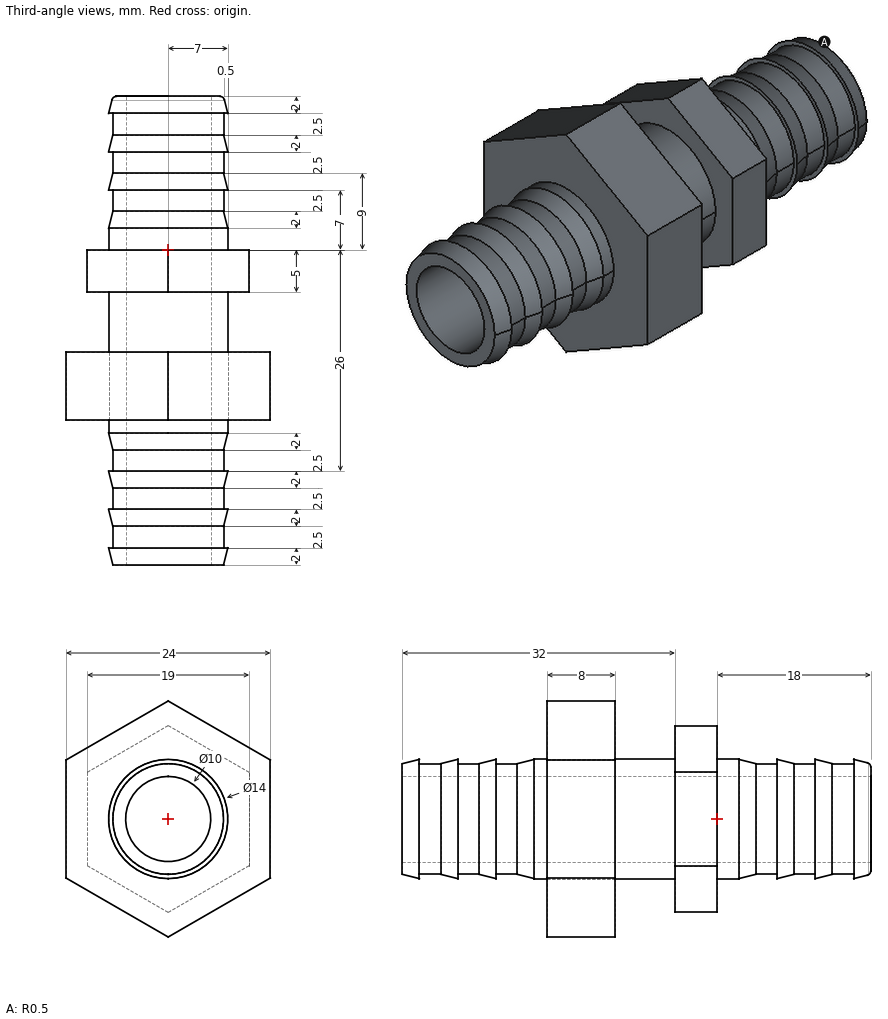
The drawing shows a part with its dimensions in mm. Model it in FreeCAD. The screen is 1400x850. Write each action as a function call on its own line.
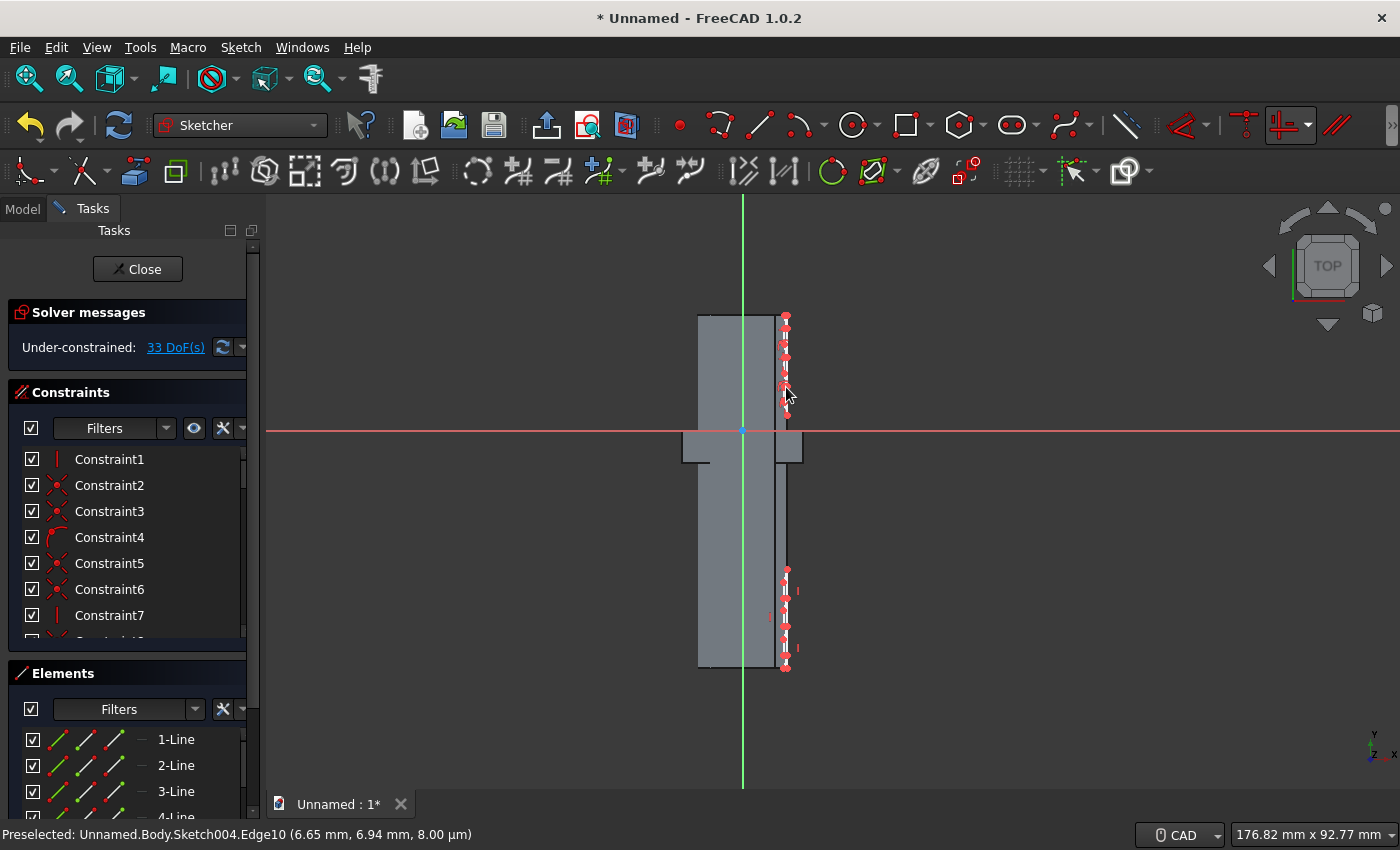
scroll(785, 599, up, 13)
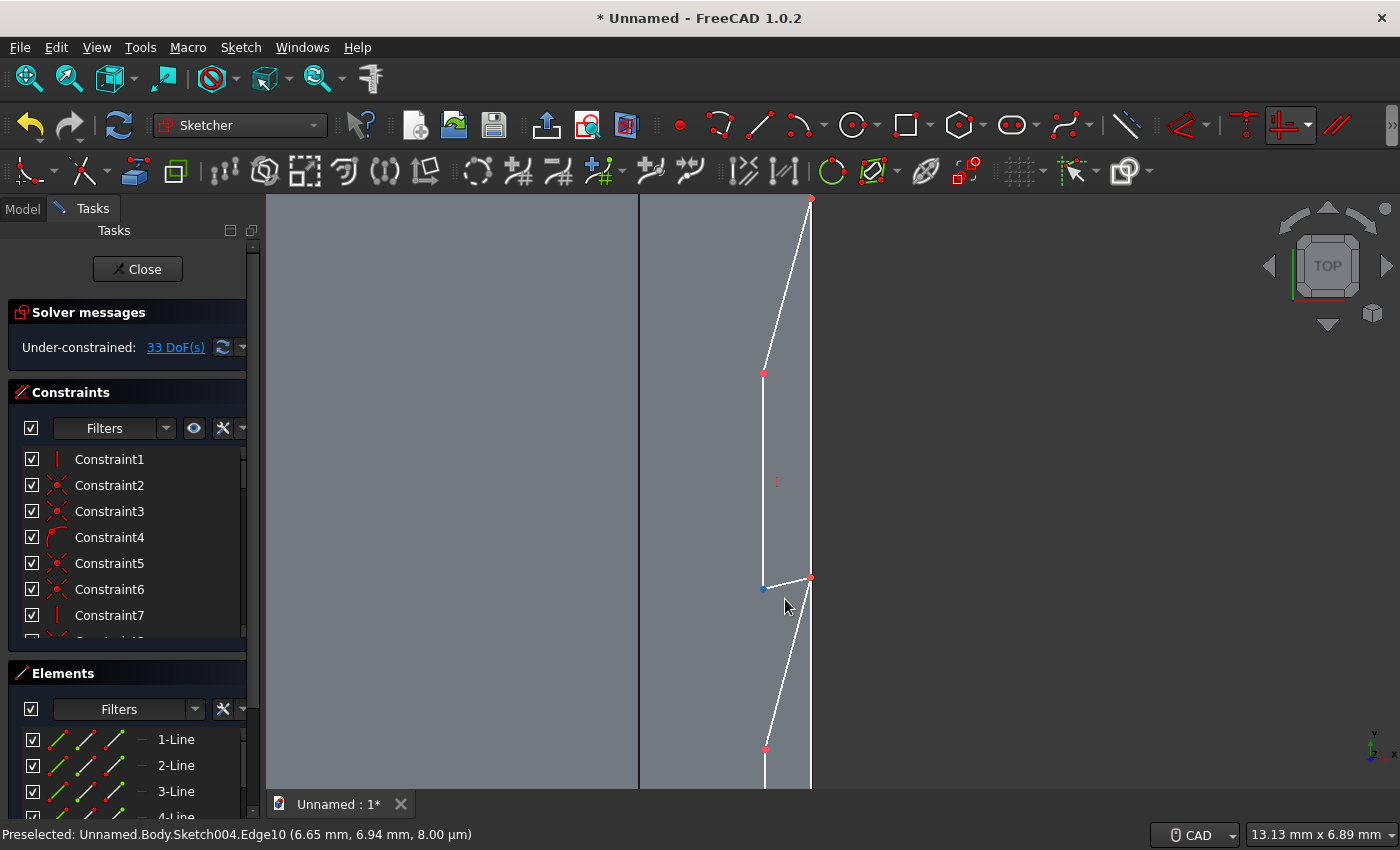
click(777, 586)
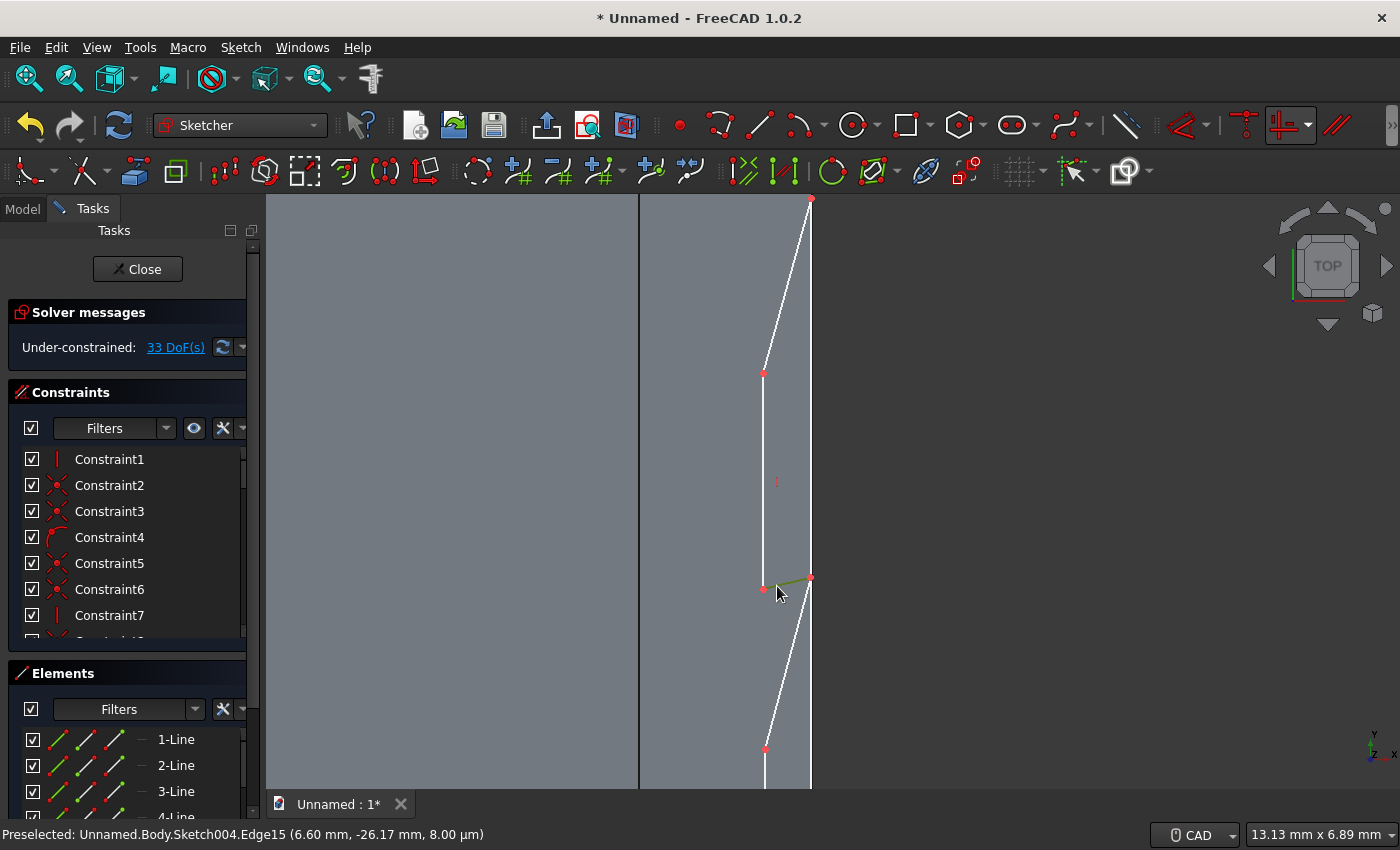
click(1310, 126)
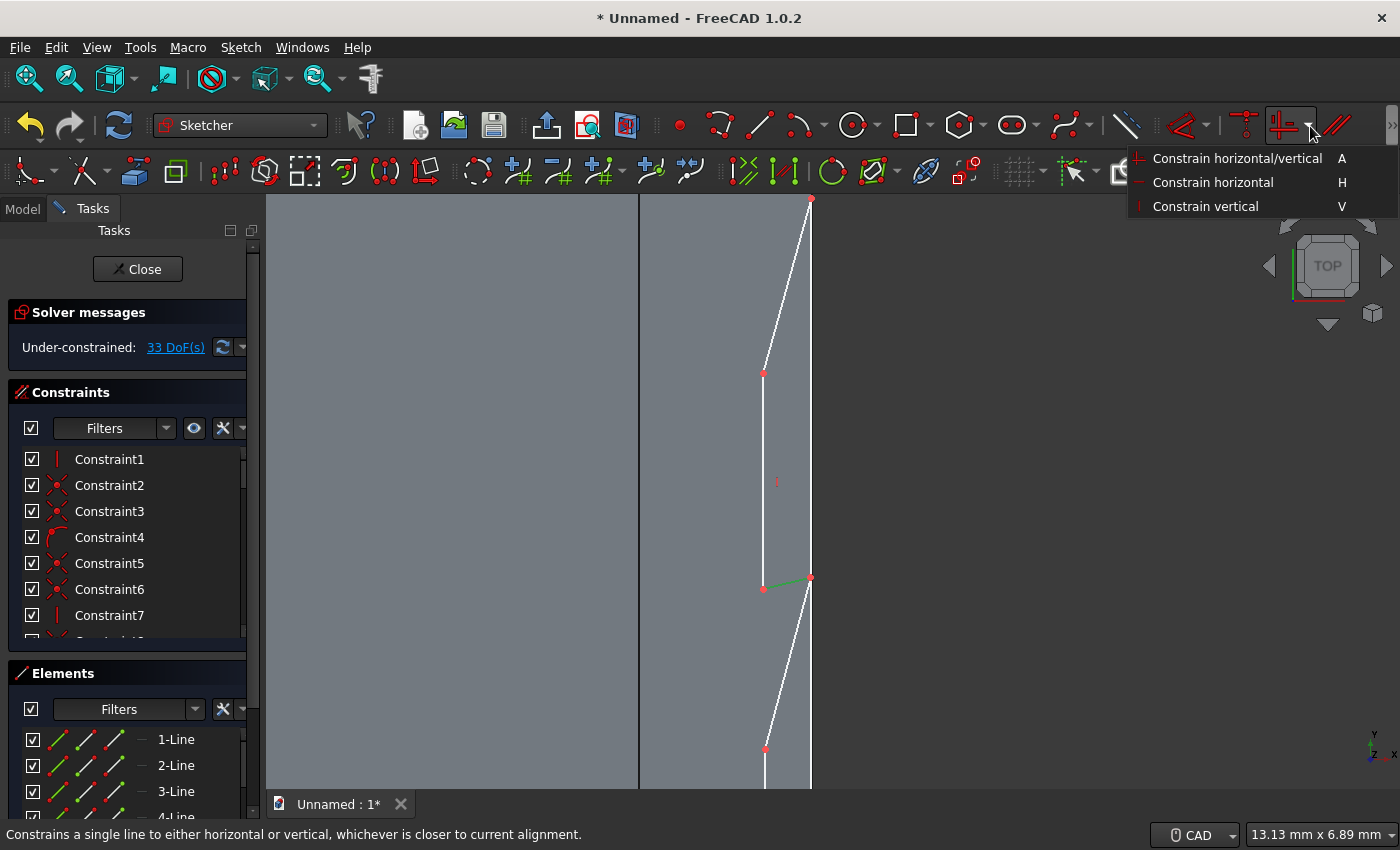
click(1263, 182)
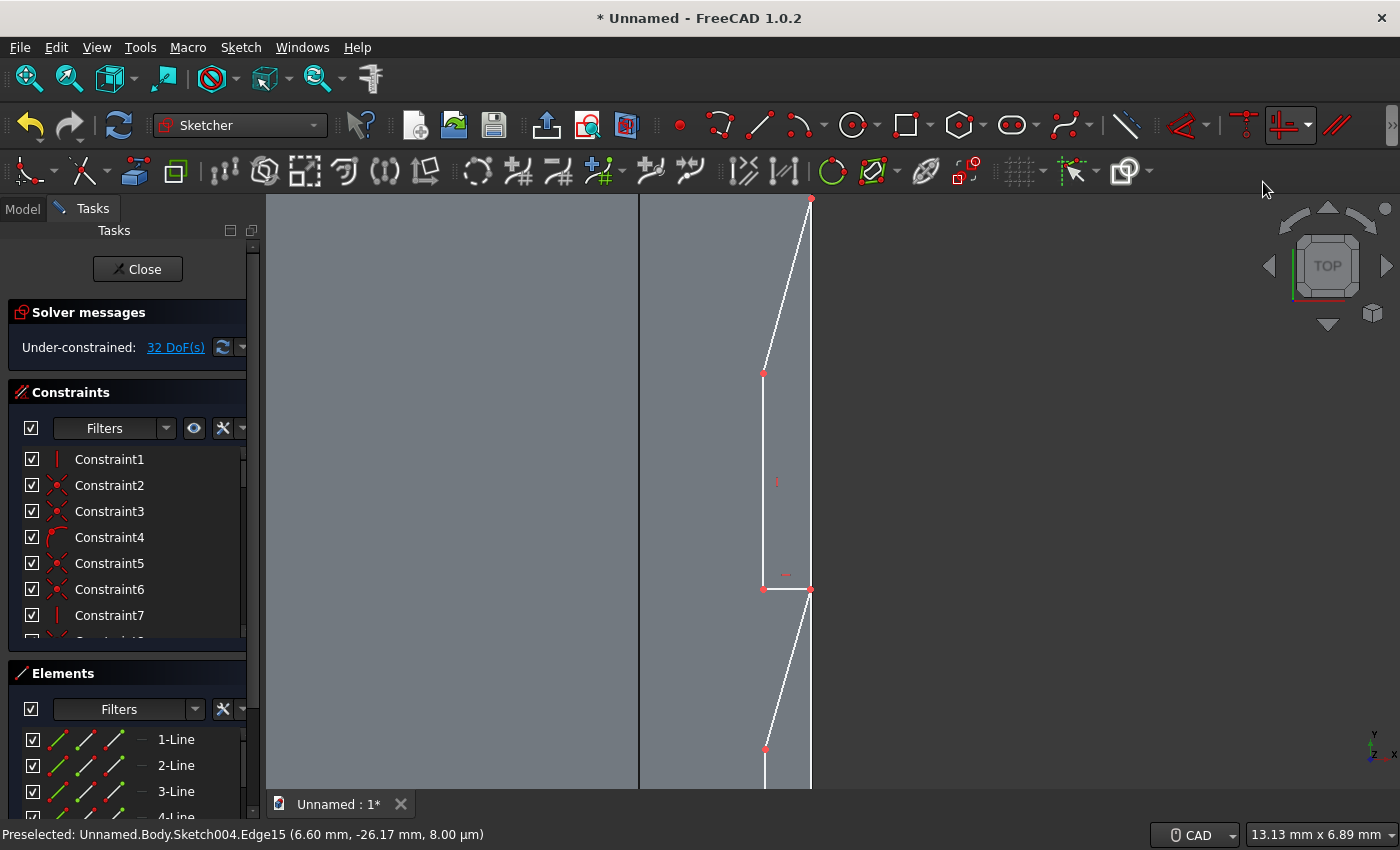
scroll(785, 599, down, 13)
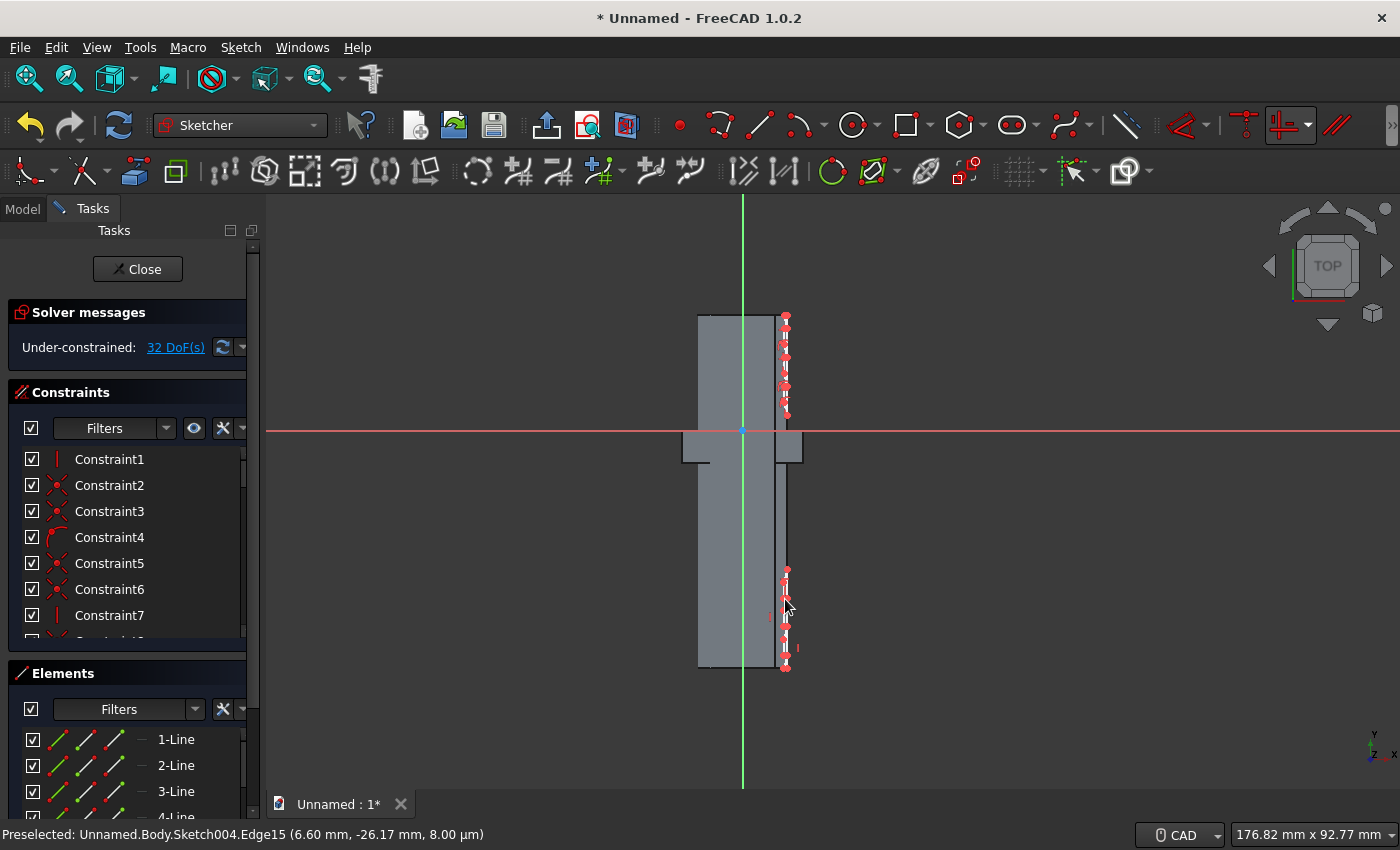
scroll(785, 627, up, 14)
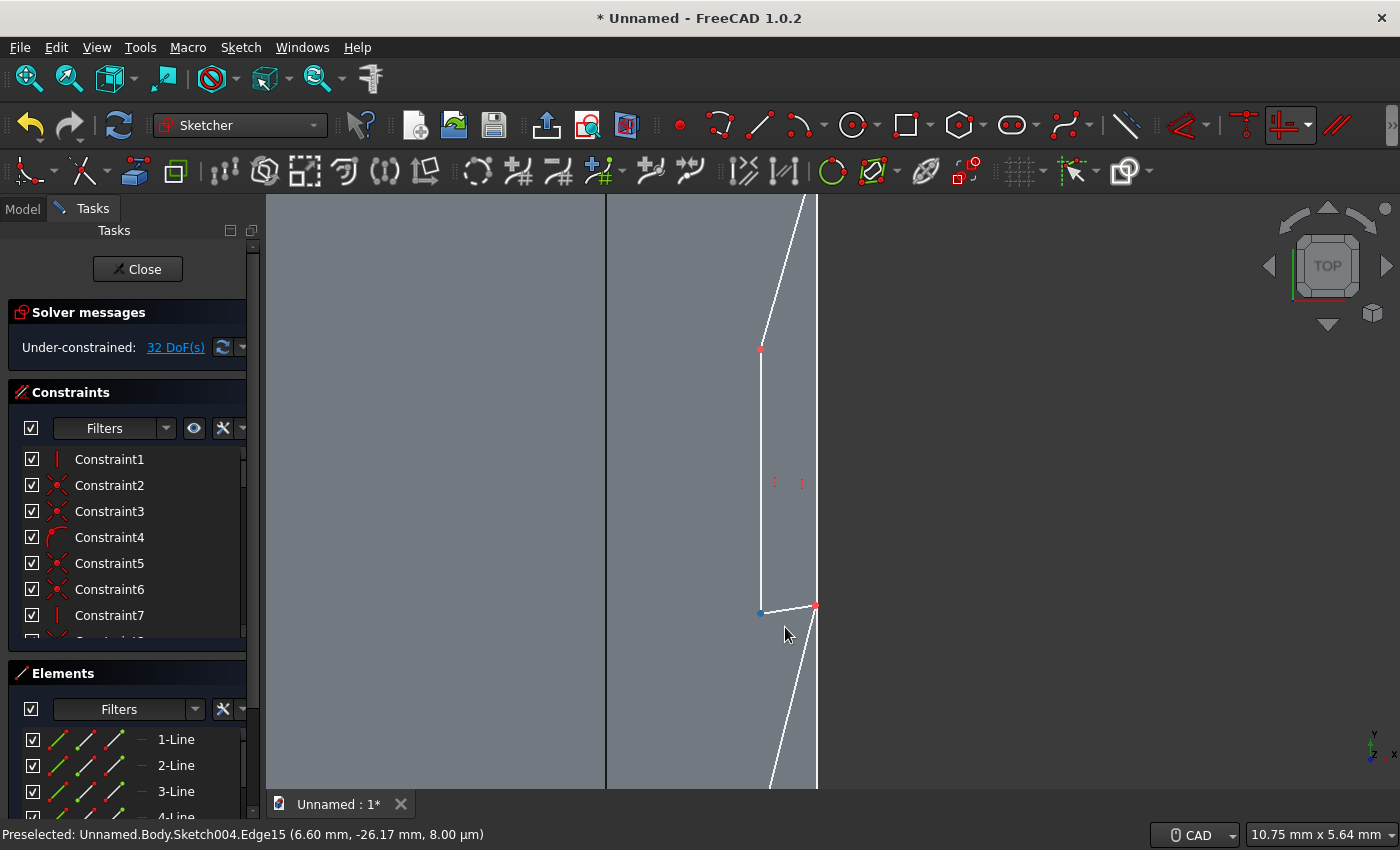
click(777, 611)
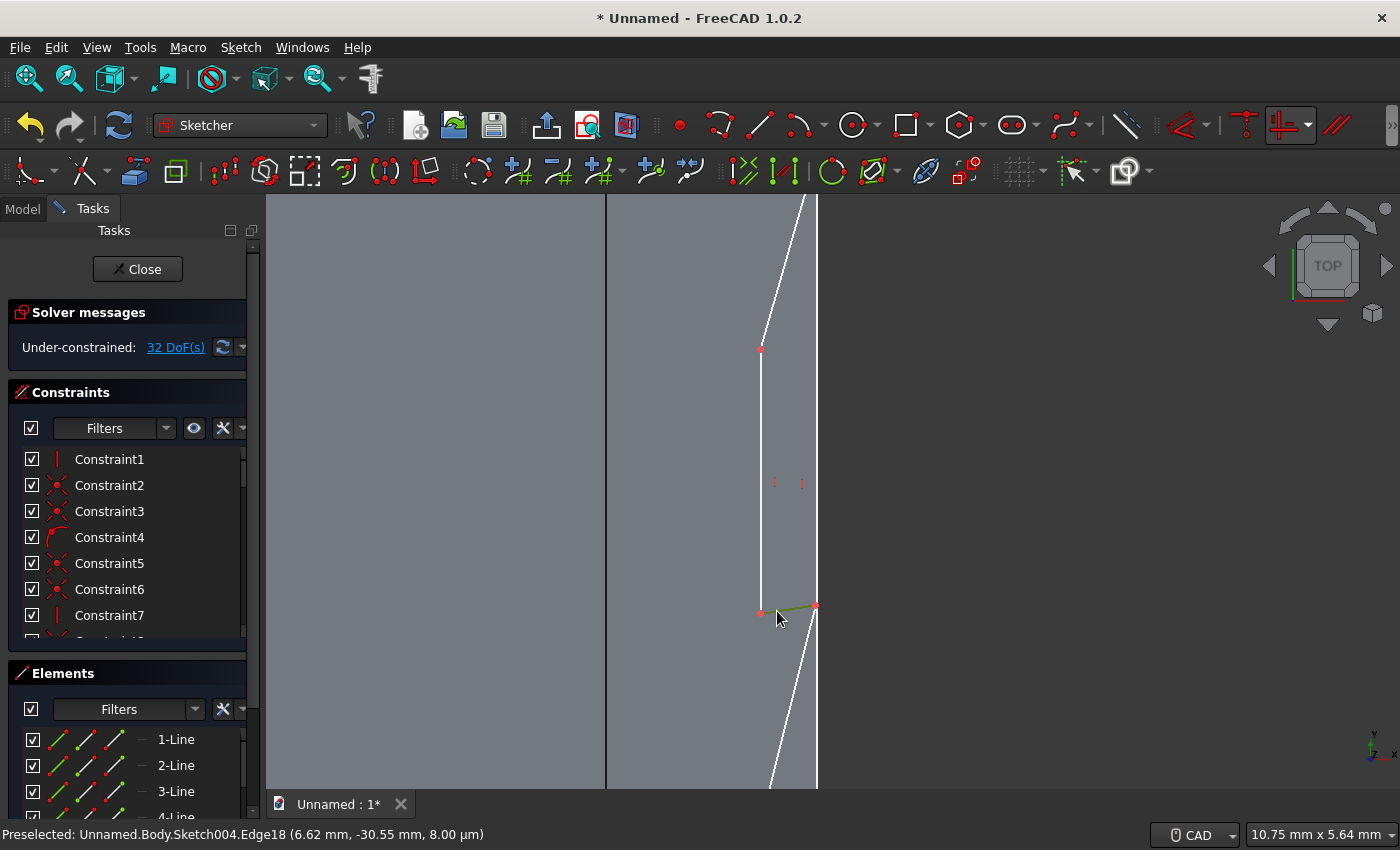
click(1310, 126)